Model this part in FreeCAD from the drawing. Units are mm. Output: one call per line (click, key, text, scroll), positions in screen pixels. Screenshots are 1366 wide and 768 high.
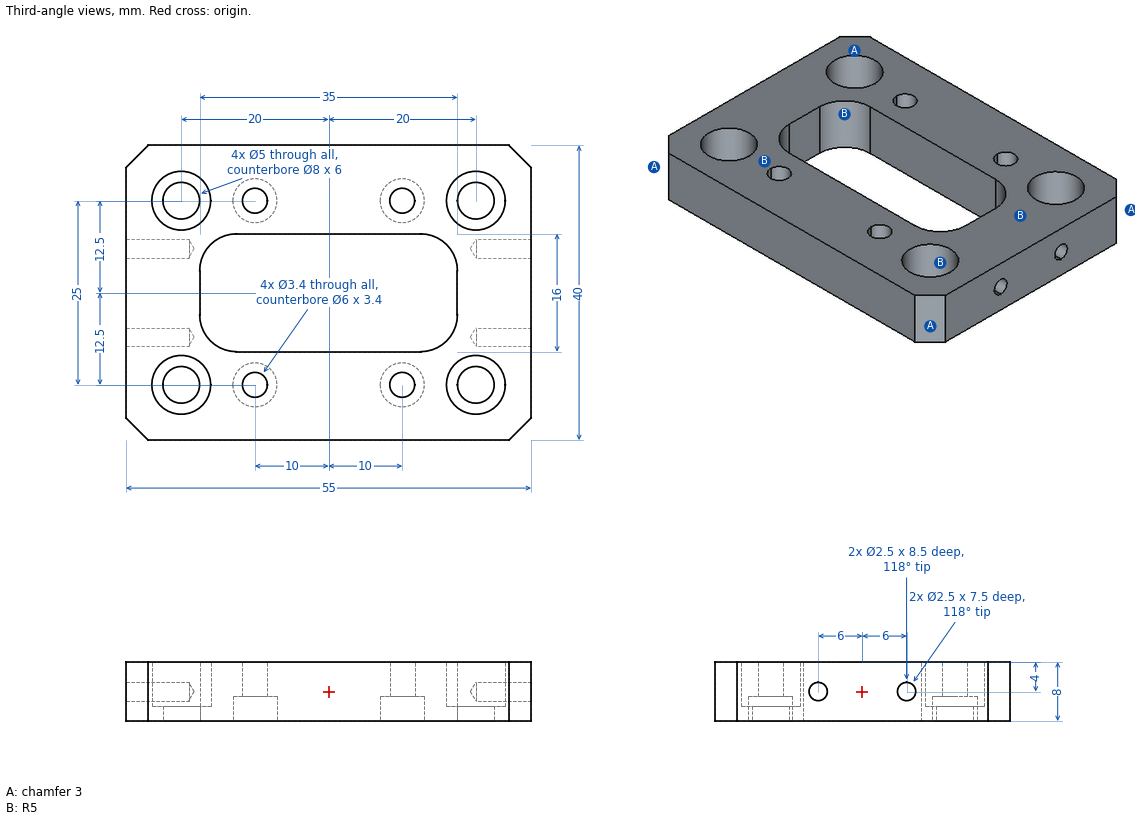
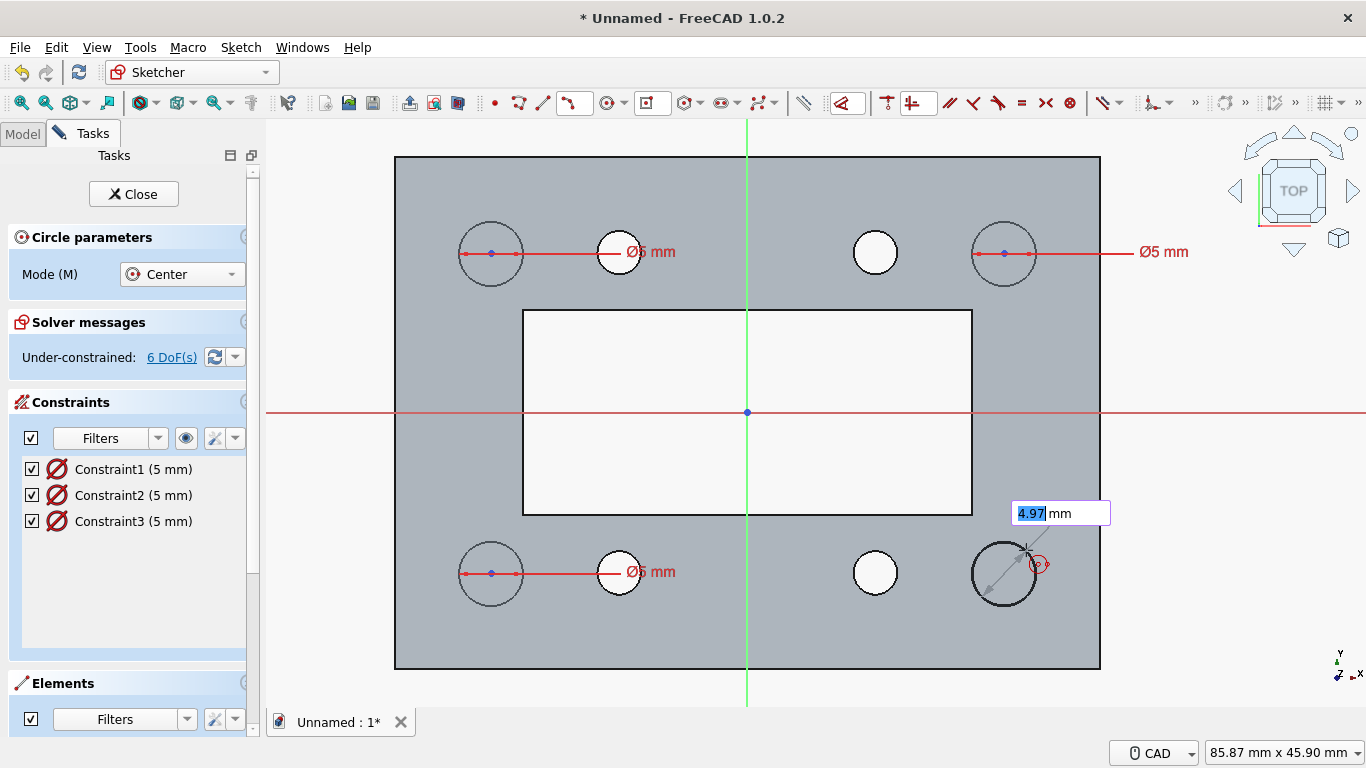
text(5)
key(Return)
key(Escape)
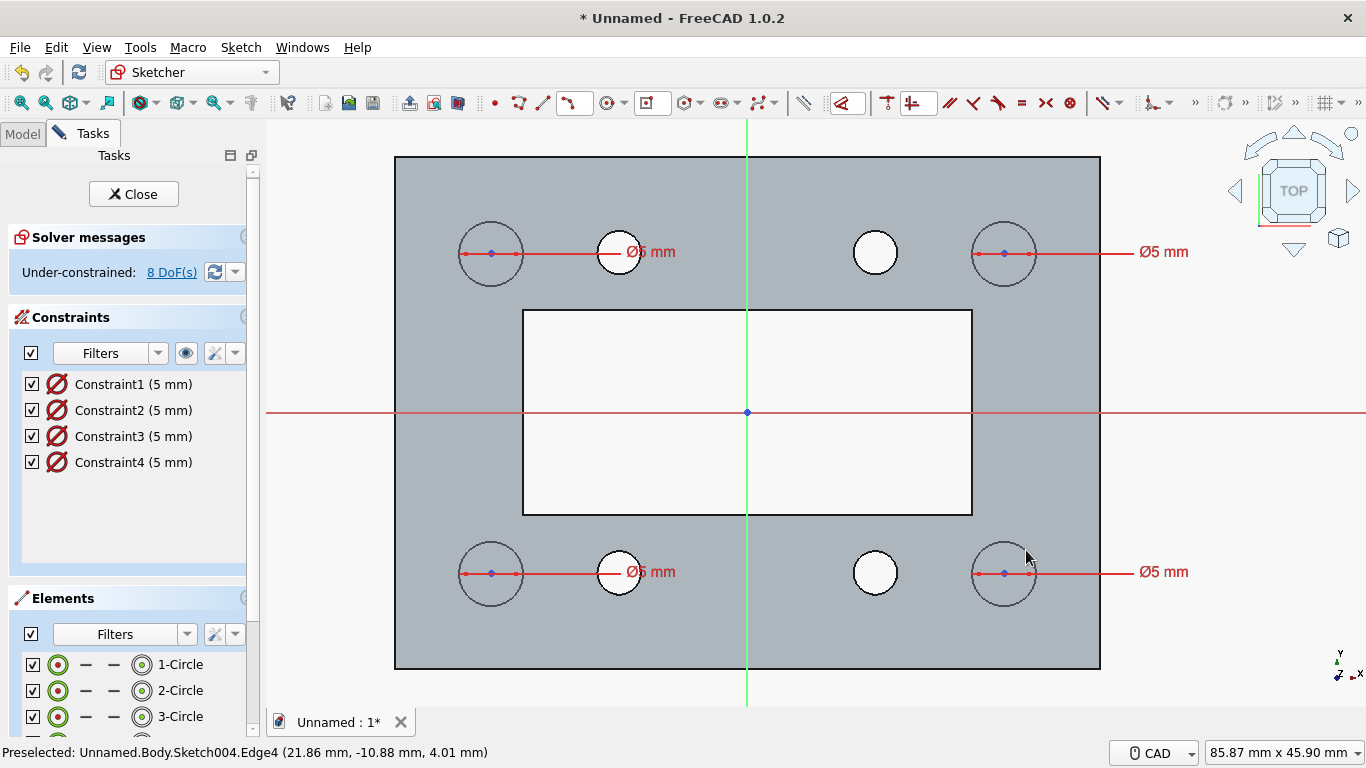
click(491, 254)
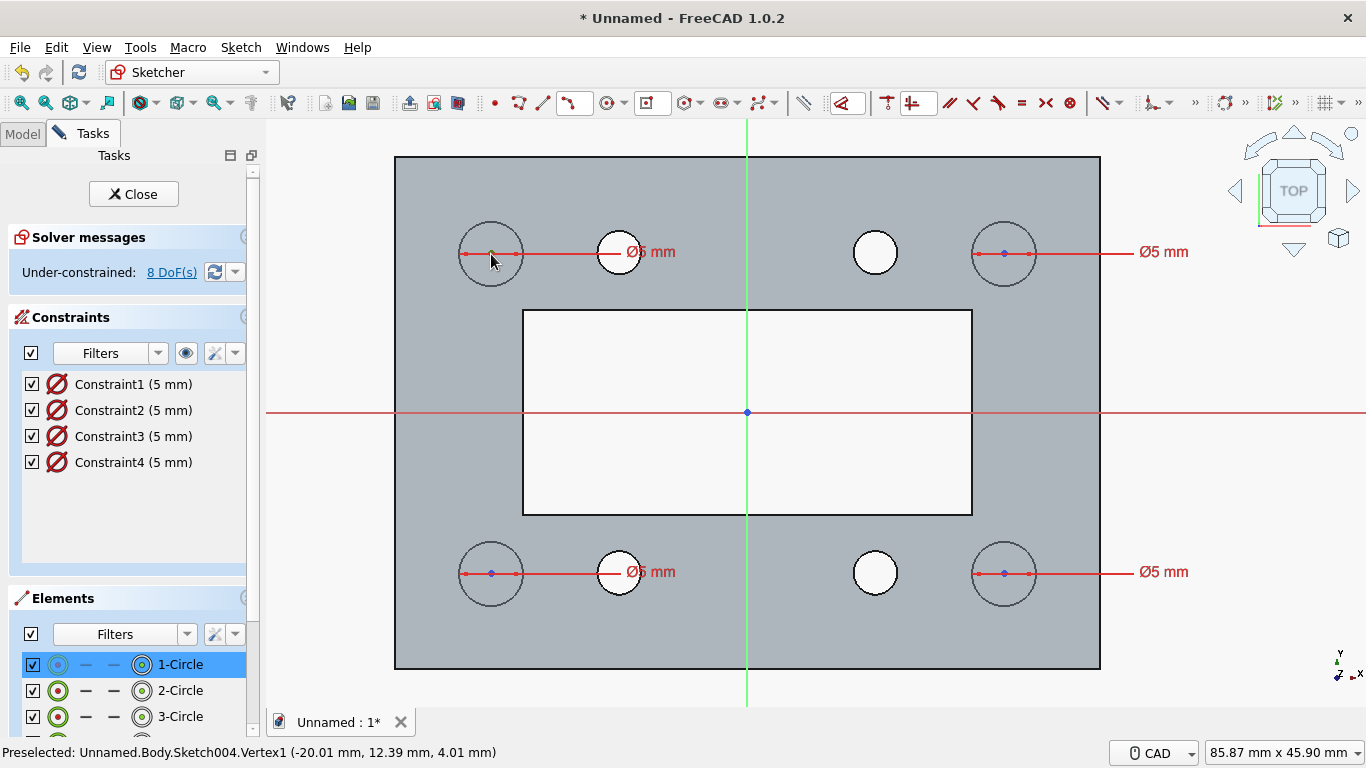
click(491, 574)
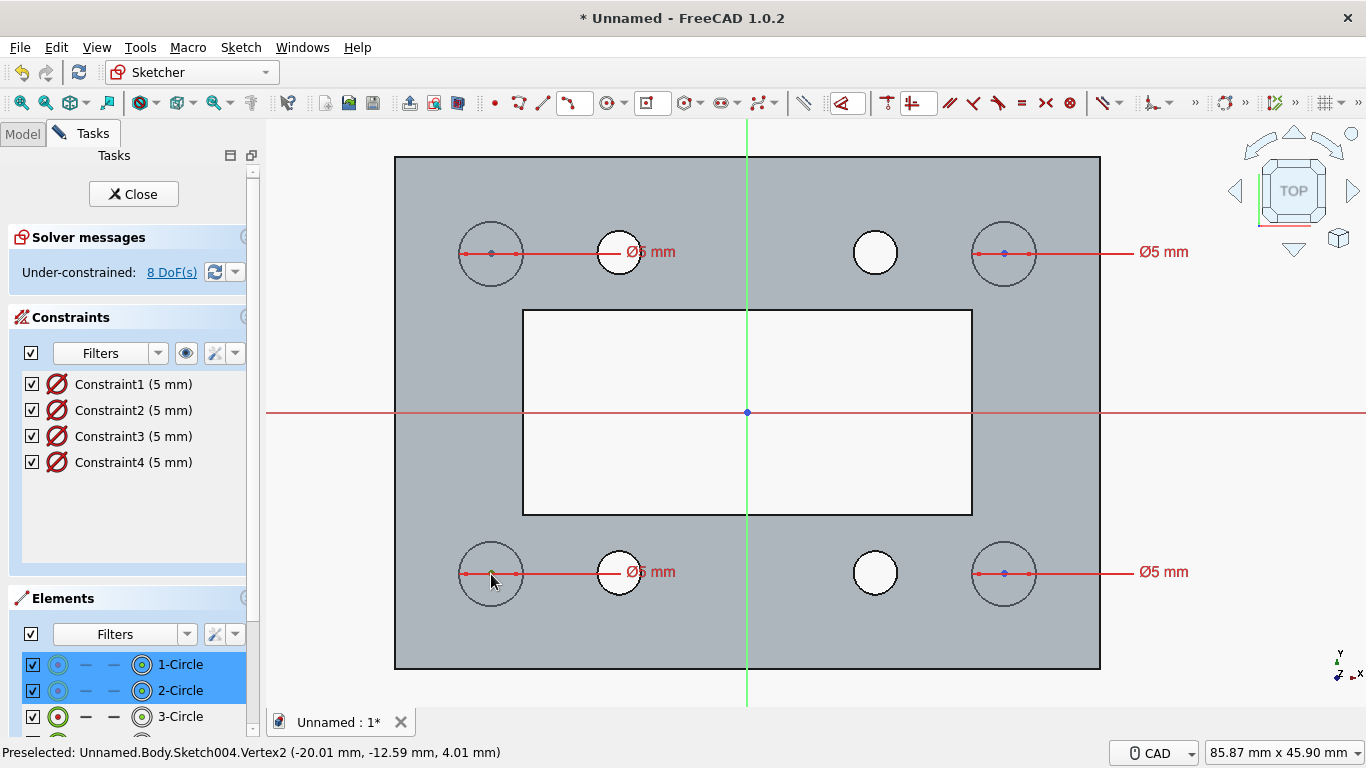
key(v)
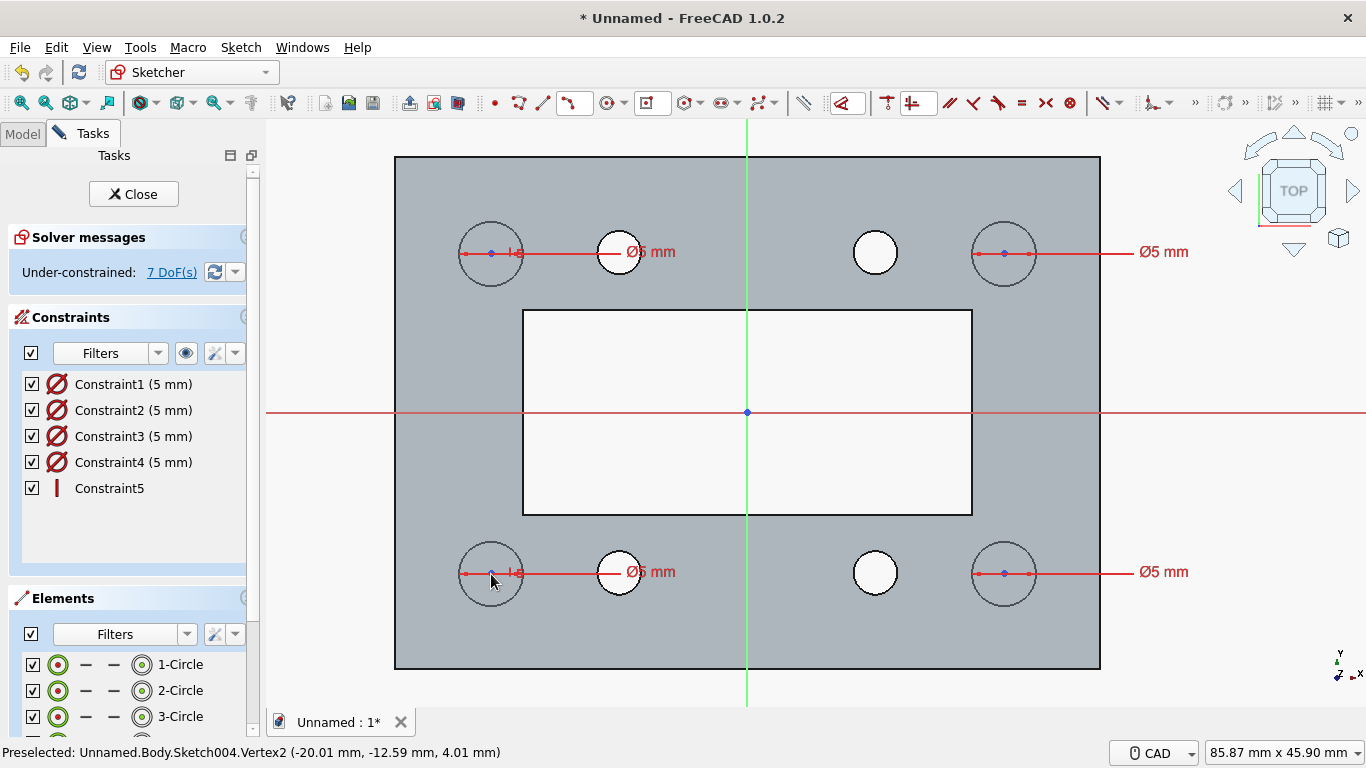
click(491, 254)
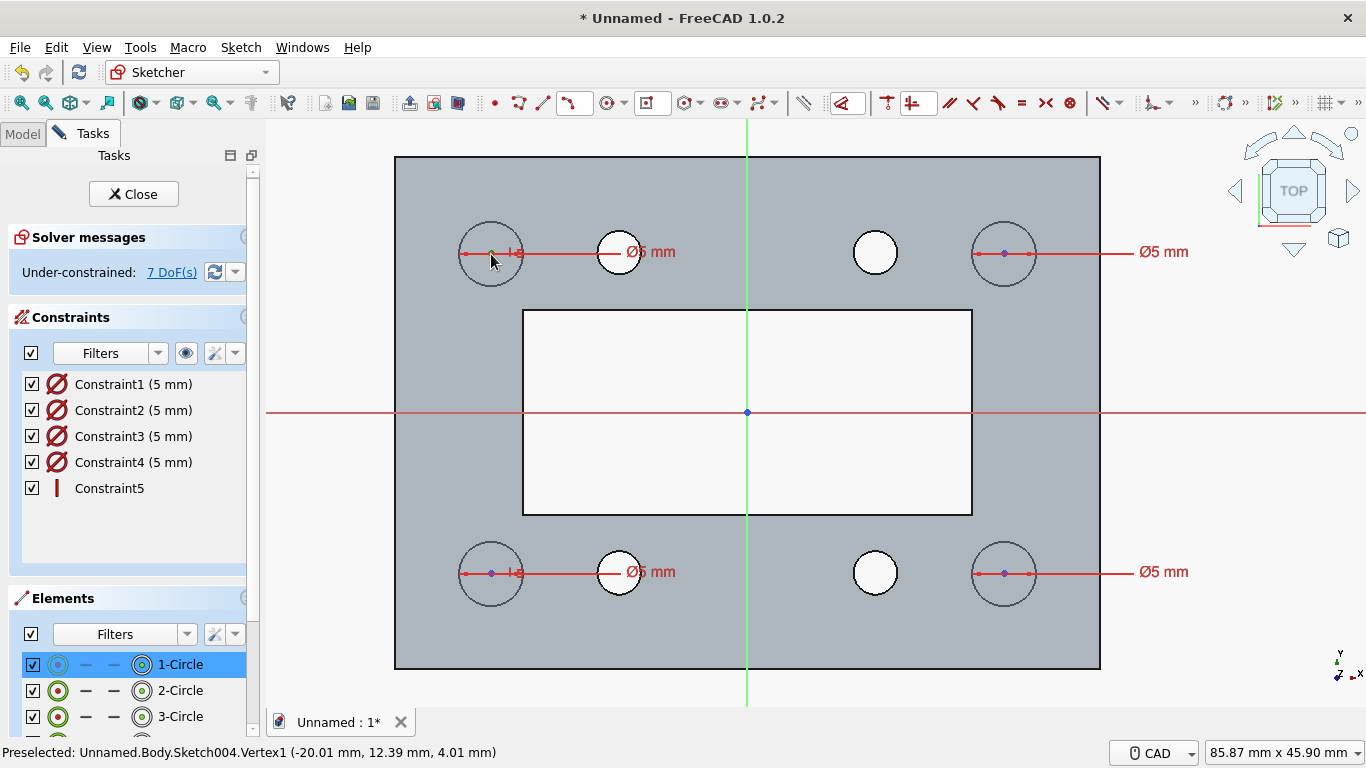
click(1004, 254)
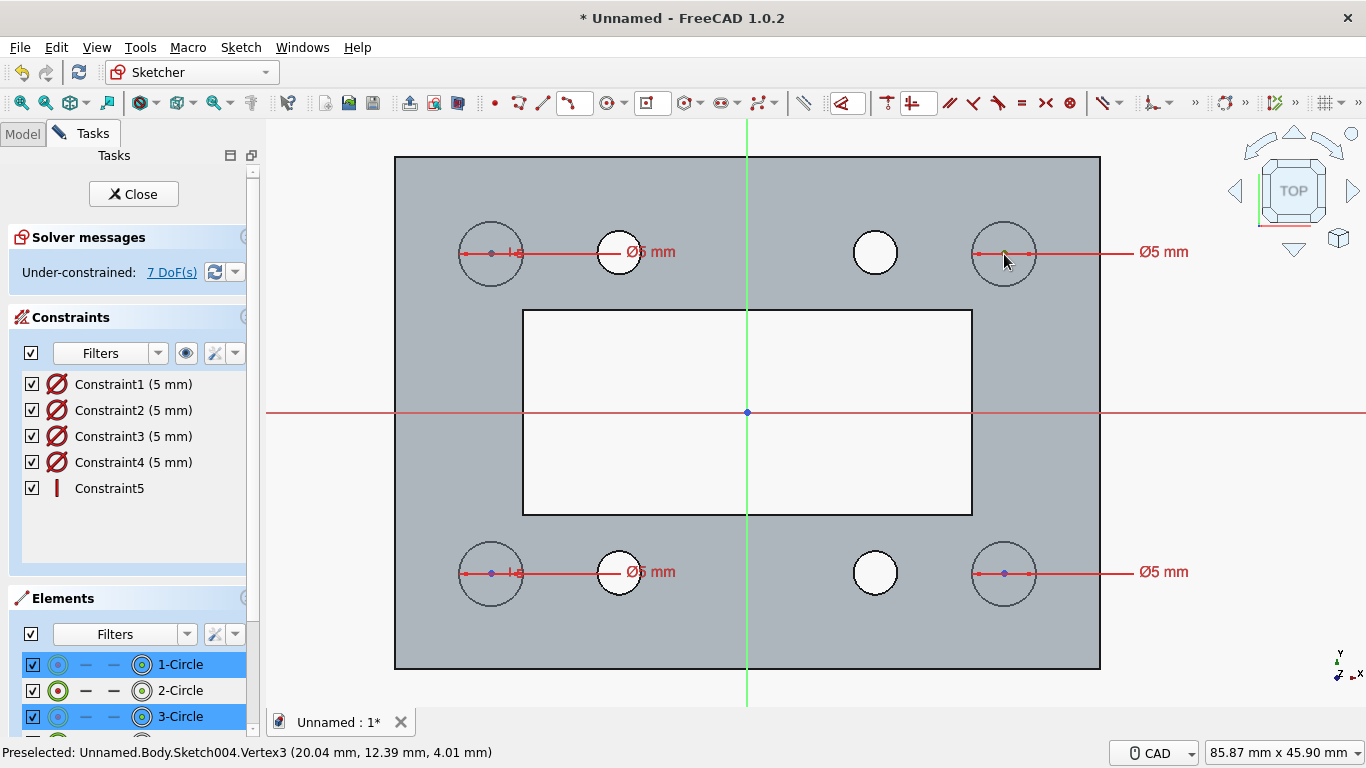
key(h)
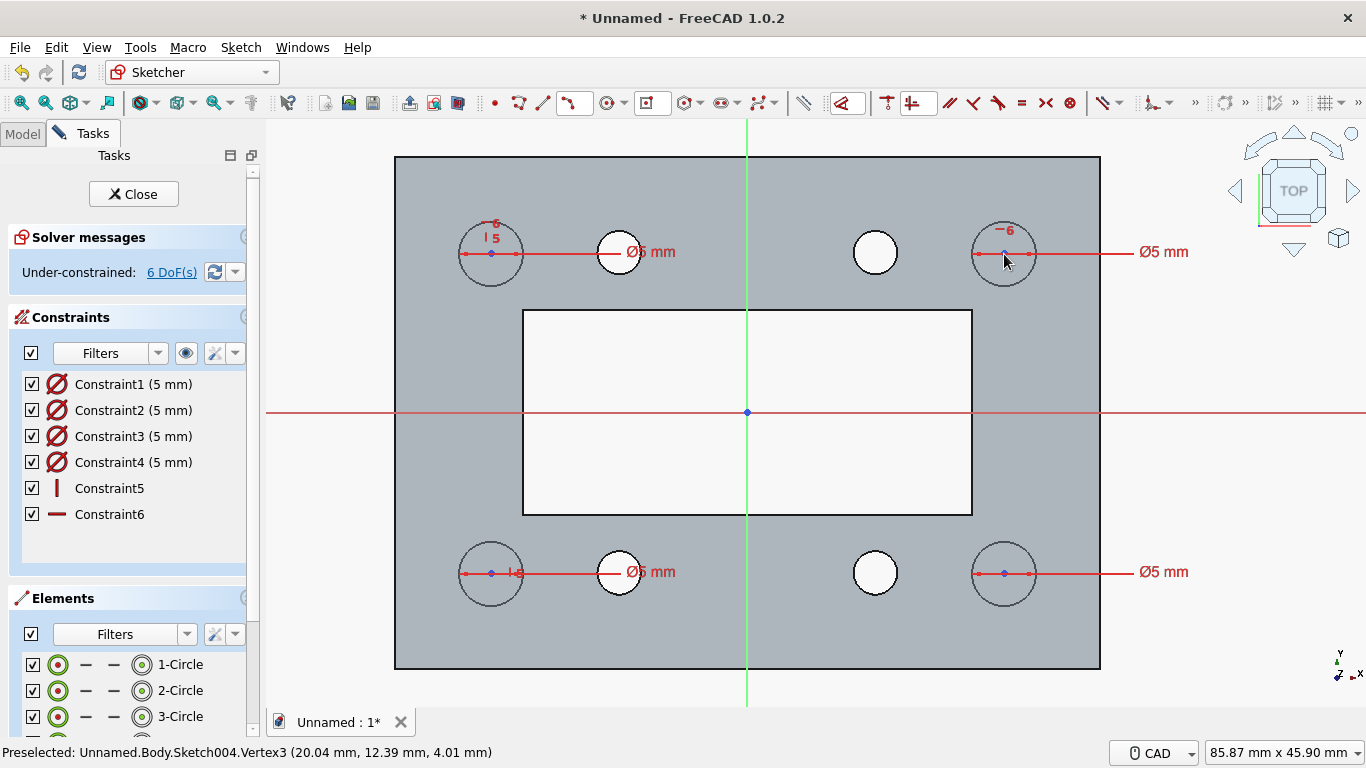
click(1004, 254)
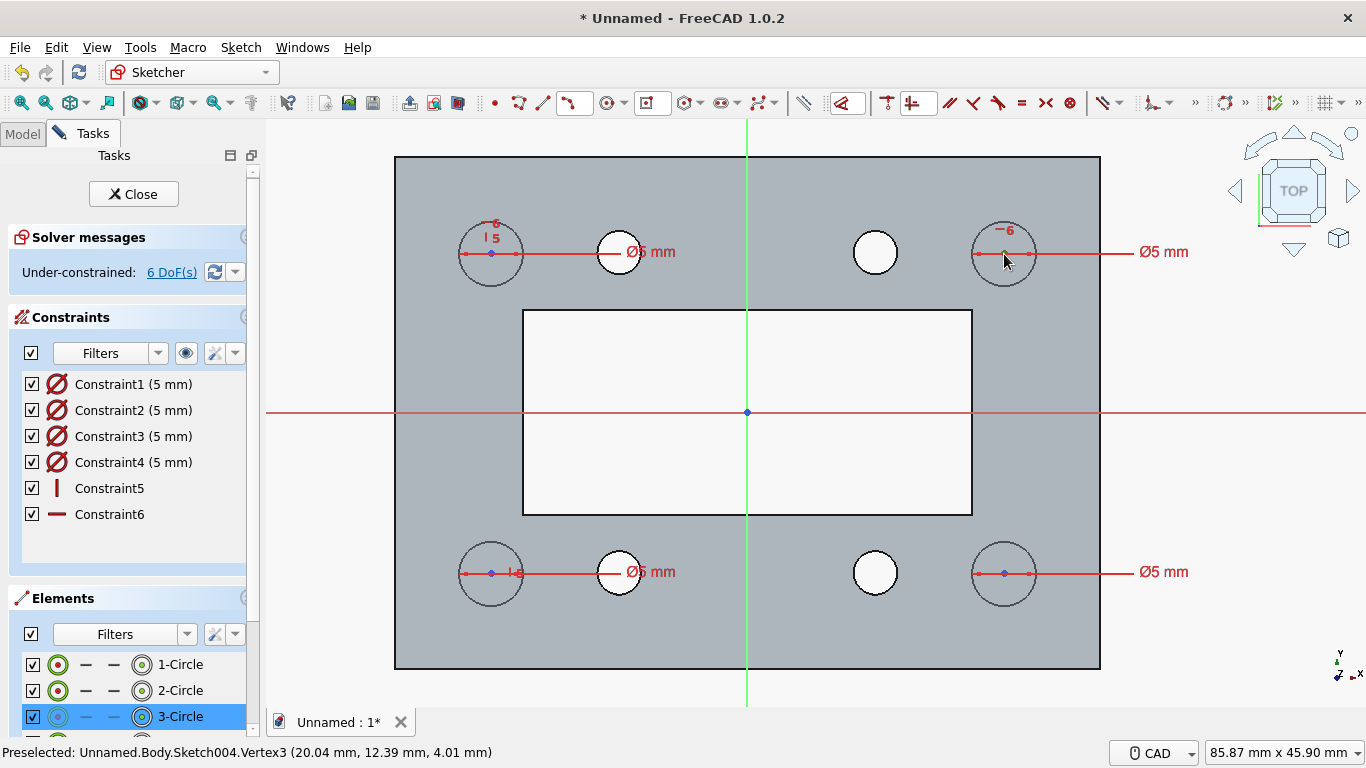
click(1004, 574)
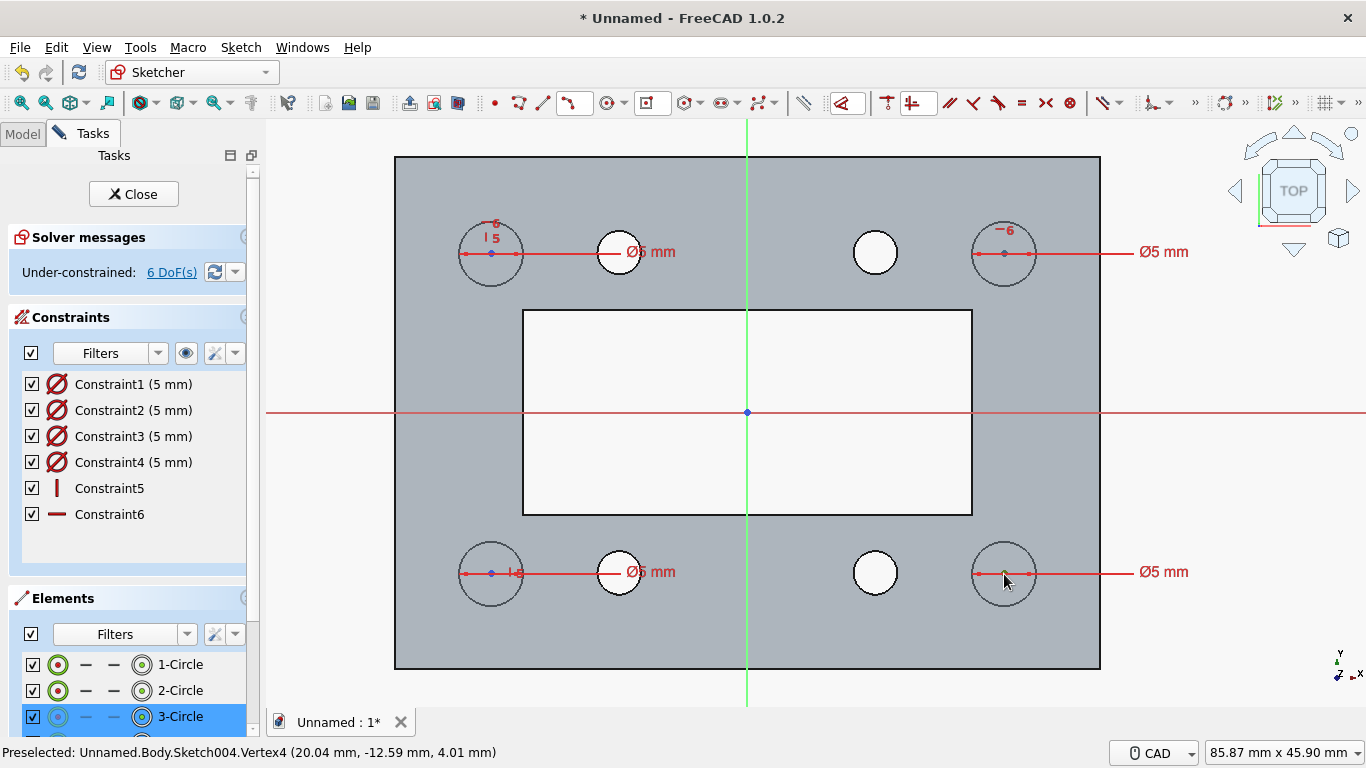
key(v)